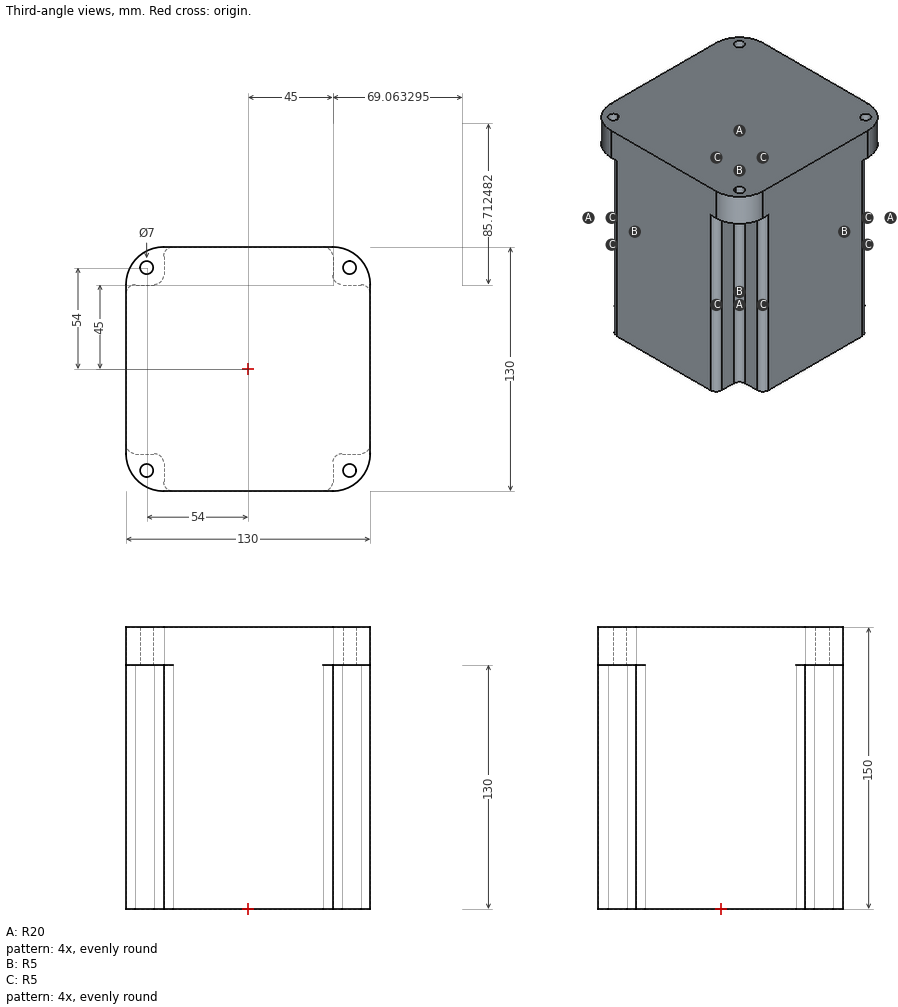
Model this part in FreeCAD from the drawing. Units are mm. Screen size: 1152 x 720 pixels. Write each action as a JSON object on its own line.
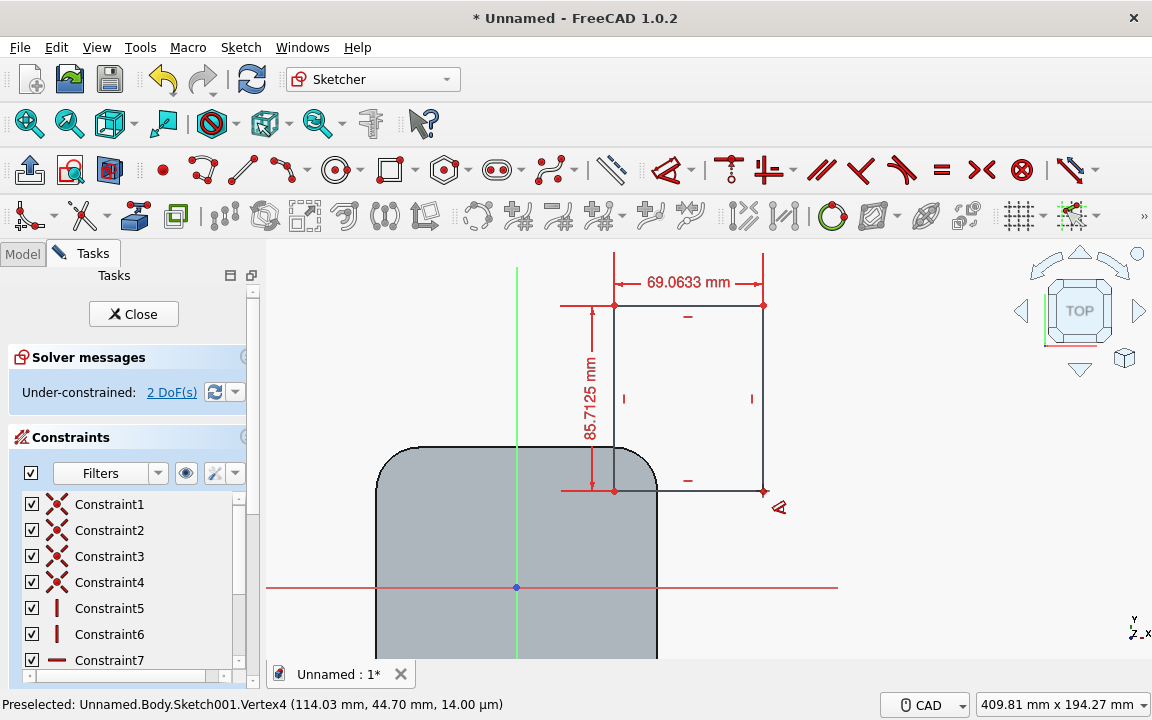
{"action": "left_click", "coordinate": [614, 306]}
{"action": "left_click", "coordinate": [565, 622]}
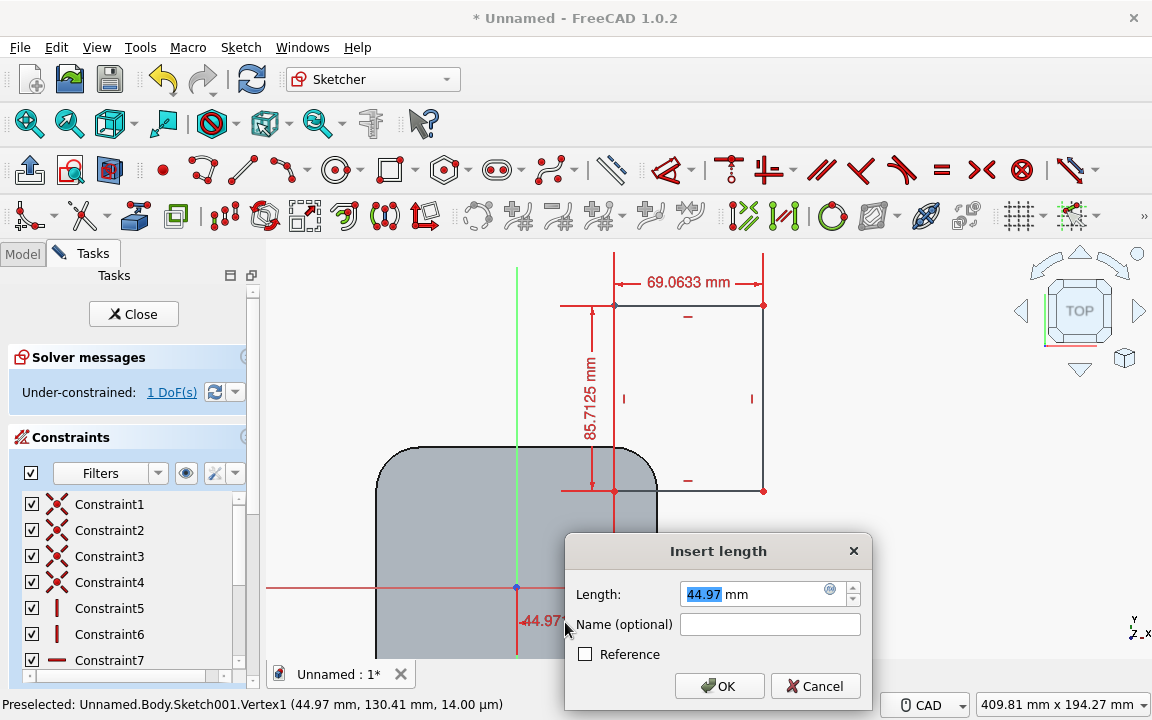
{"action": "type", "text": "45"}
{"action": "key", "text": "Return"}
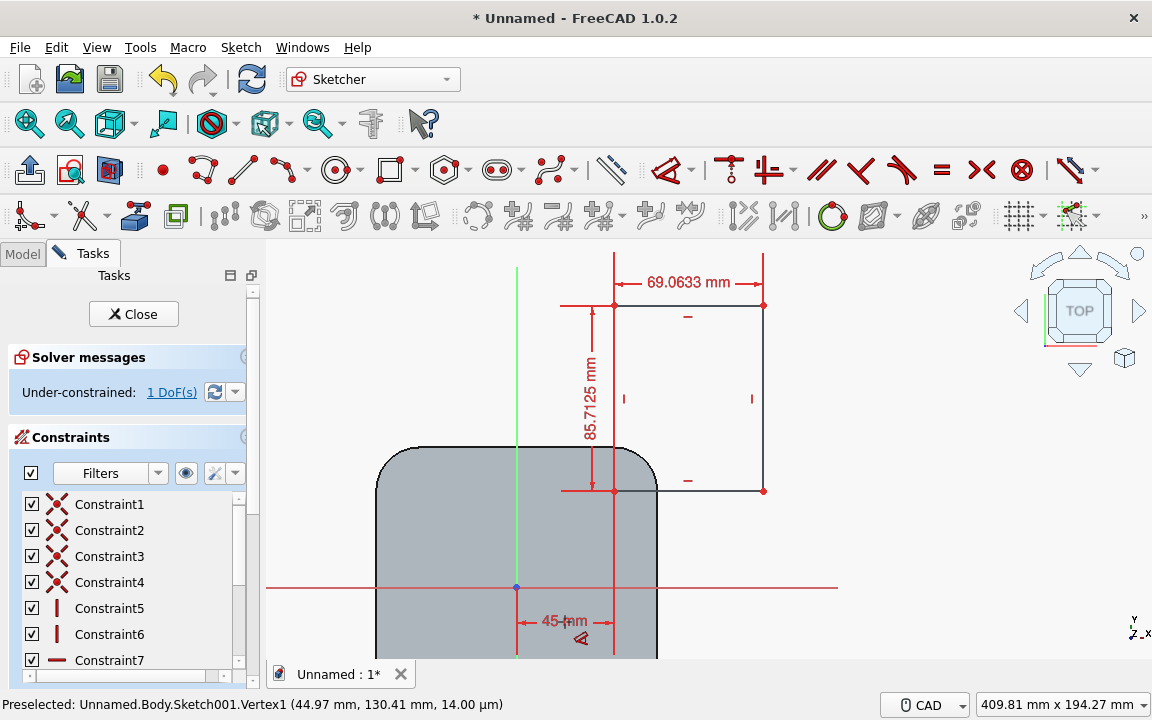
{"action": "left_click", "coordinate": [614, 491]}
{"action": "left_click", "coordinate": [483, 540]}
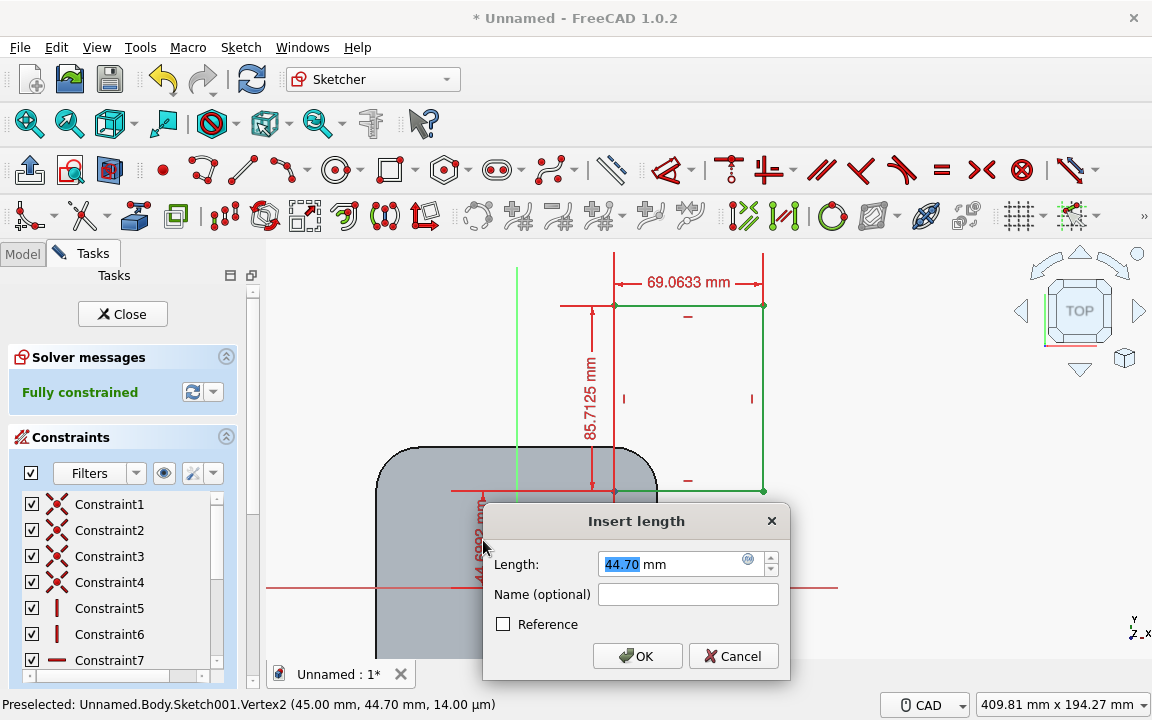
{"action": "type", "text": "45"}
{"action": "key", "text": "Return"}
{"action": "key", "text": "Escape"}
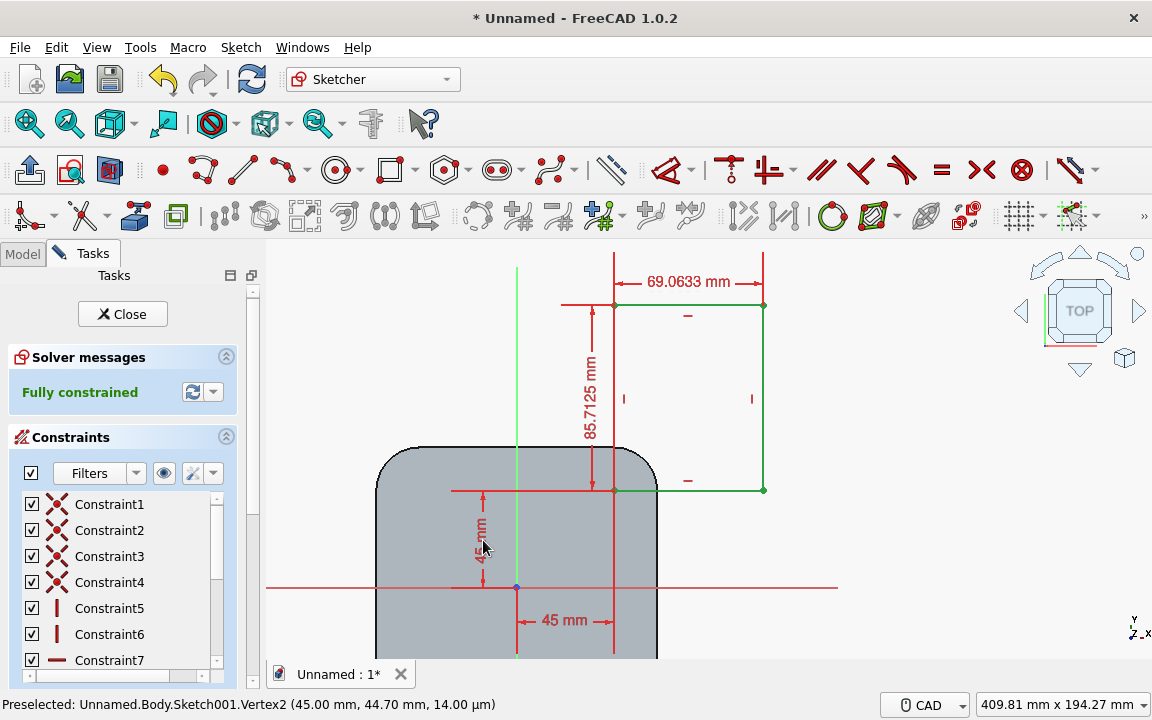
{"action": "left_click", "coordinate": [123, 314]}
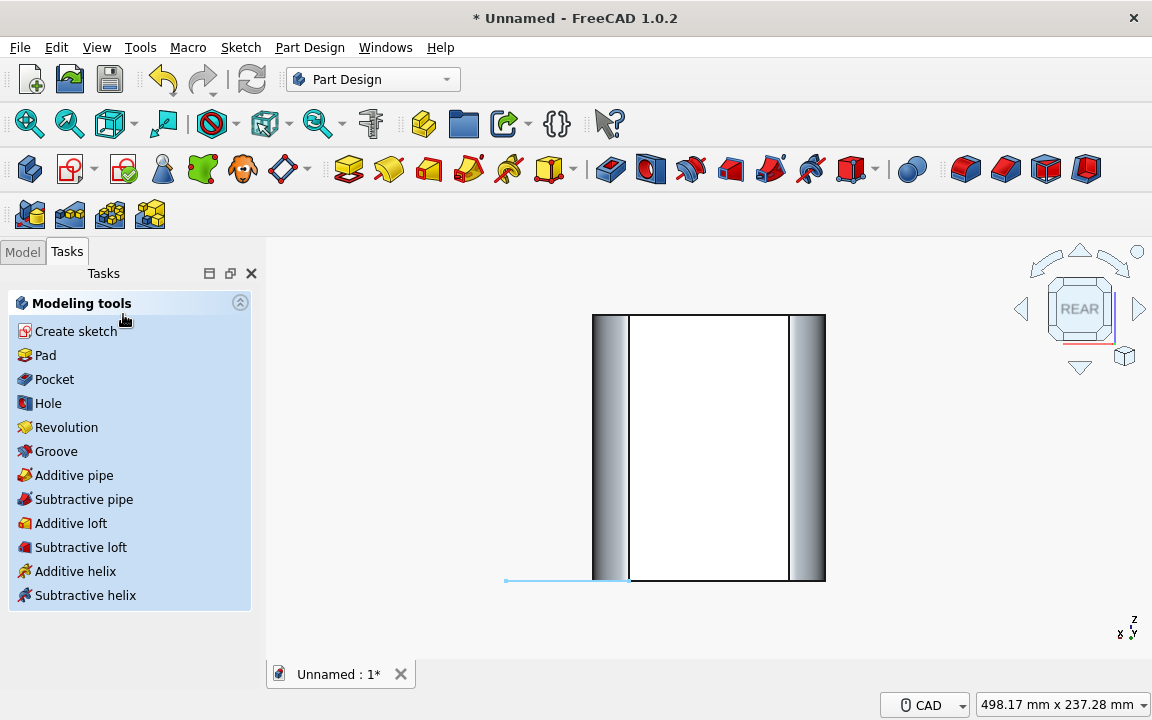
{"action": "left_click", "coordinate": [612, 170]}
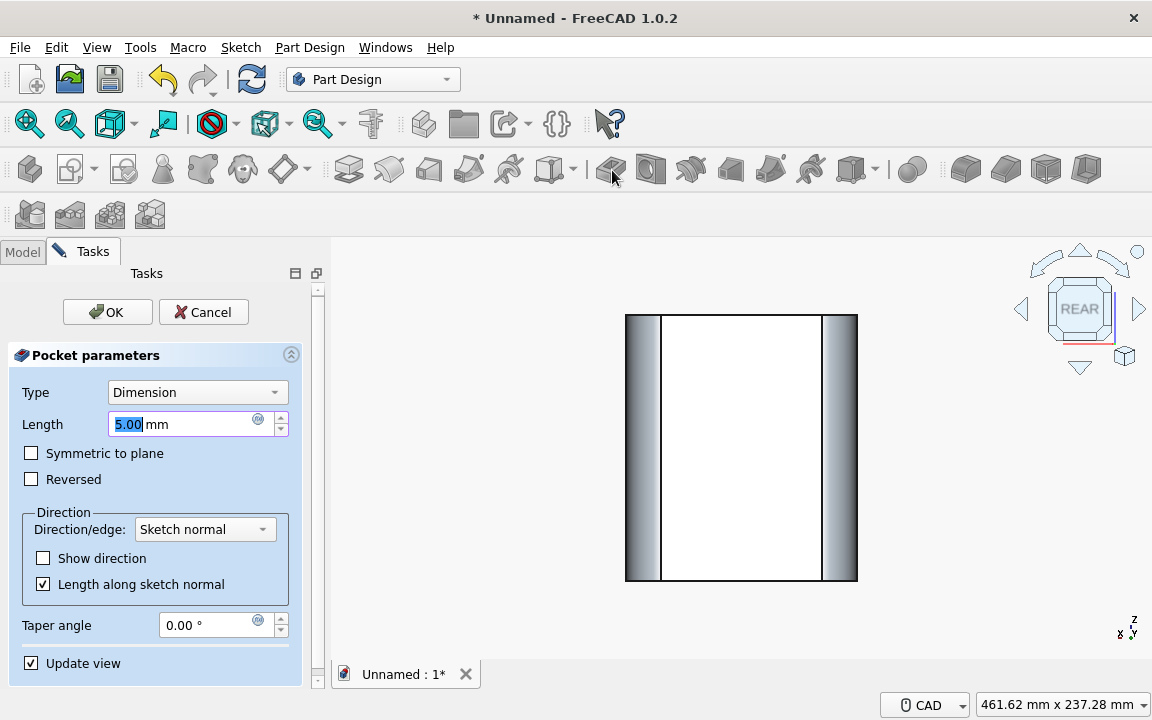
{"action": "type", "text": "130"}
{"action": "key", "text": "Tab"}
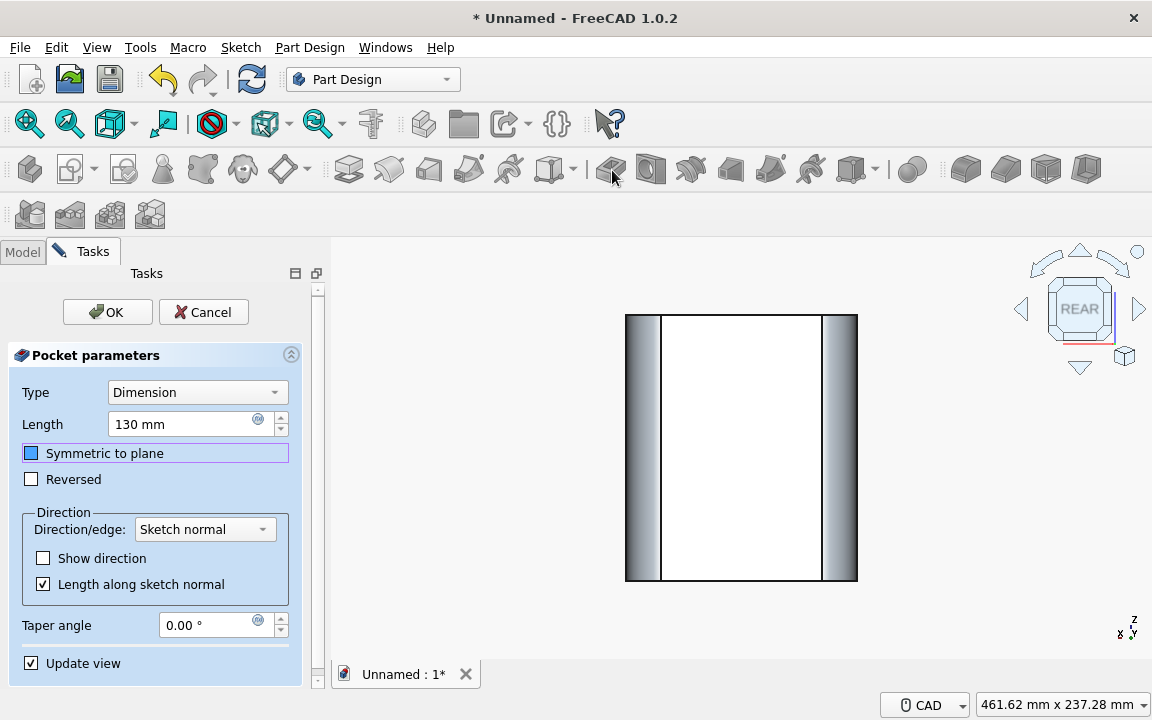
{"action": "left_click", "coordinate": [30, 479]}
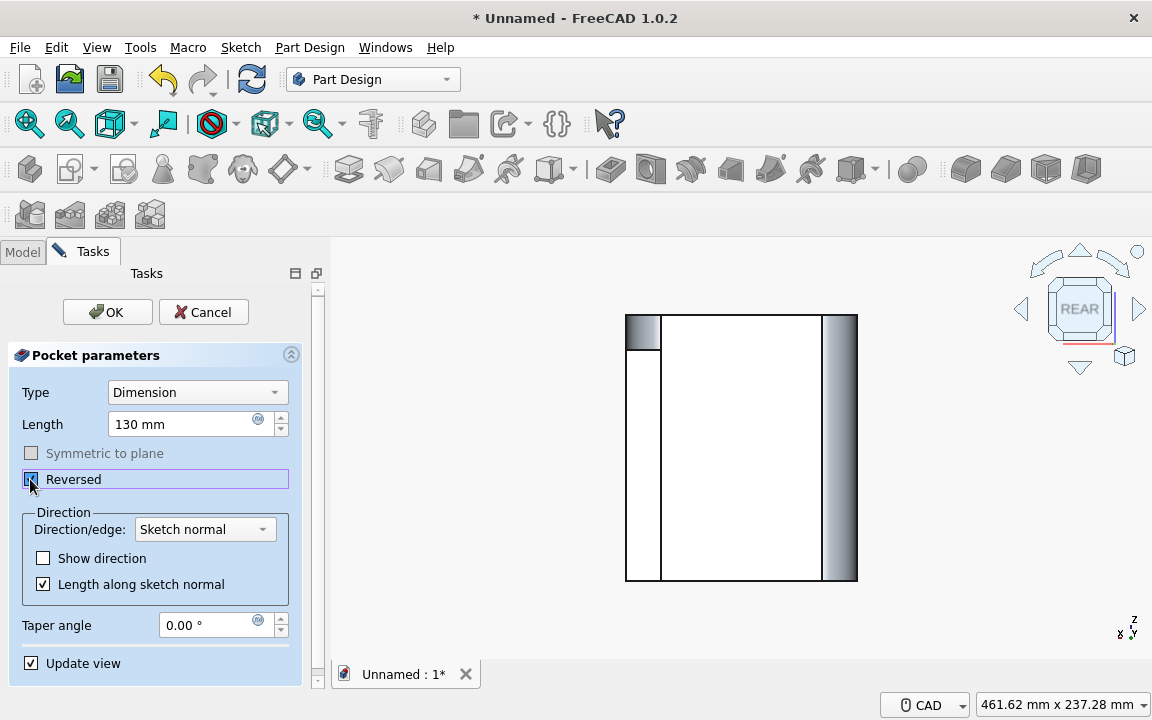
{"action": "left_click", "coordinate": [108, 312]}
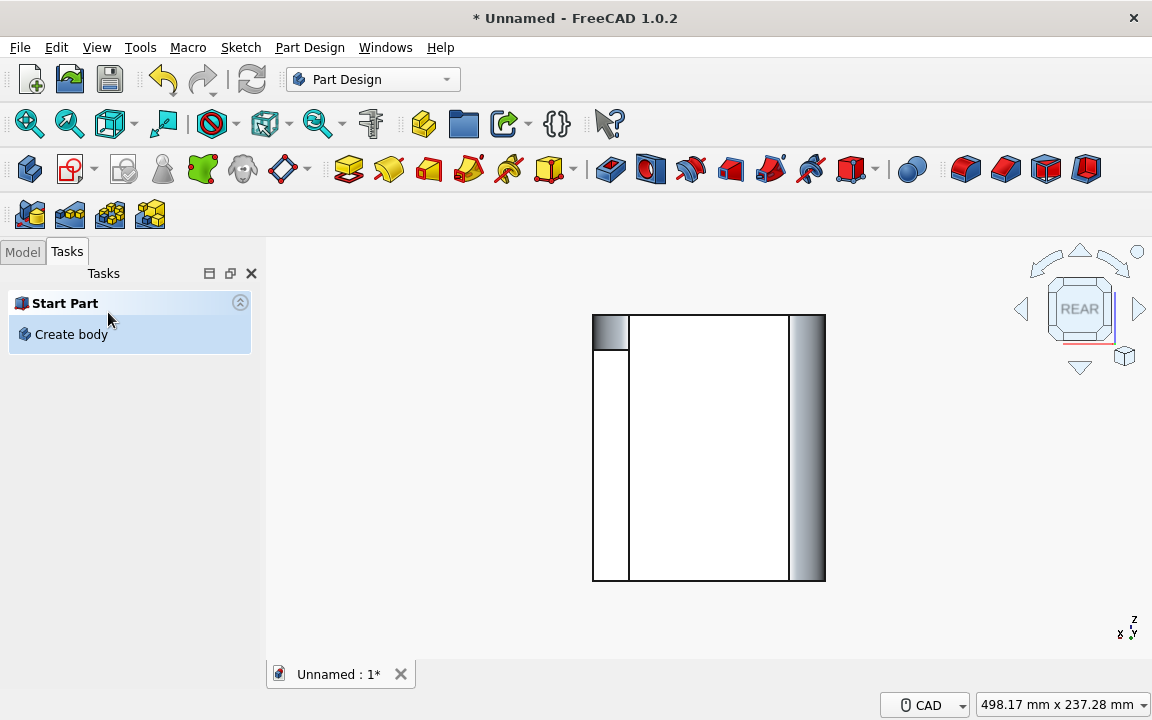
{"action": "left_click", "coordinate": [23, 251]}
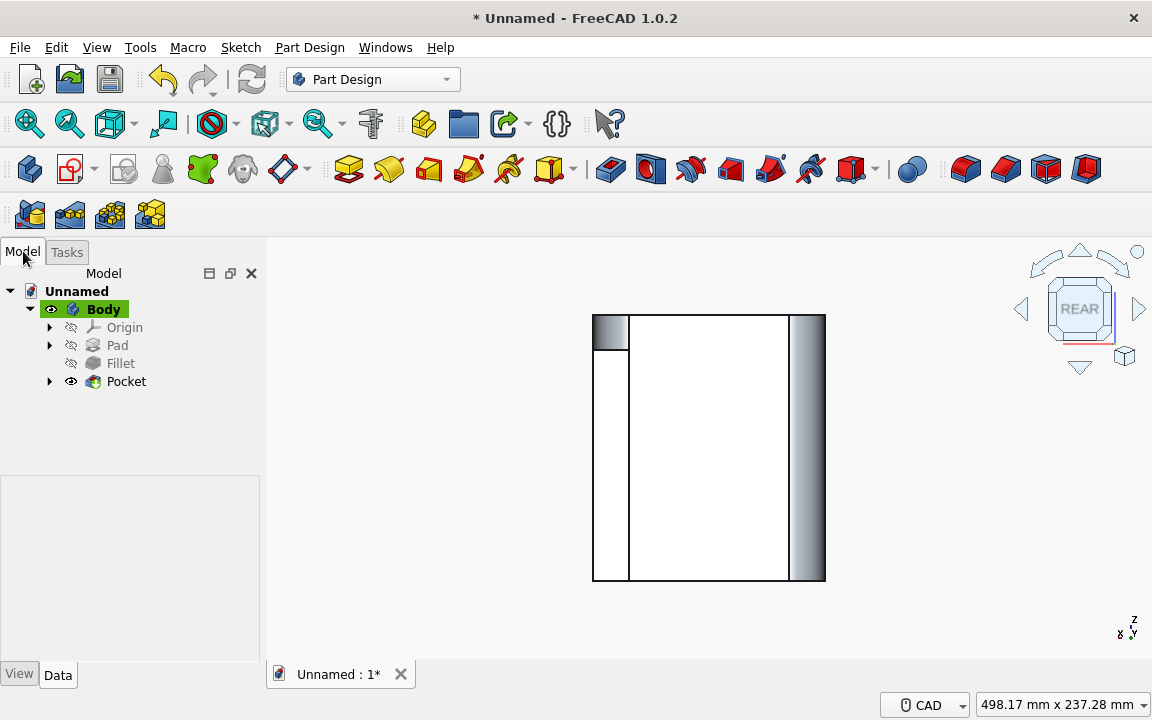
{"action": "left_click", "coordinate": [116, 381]}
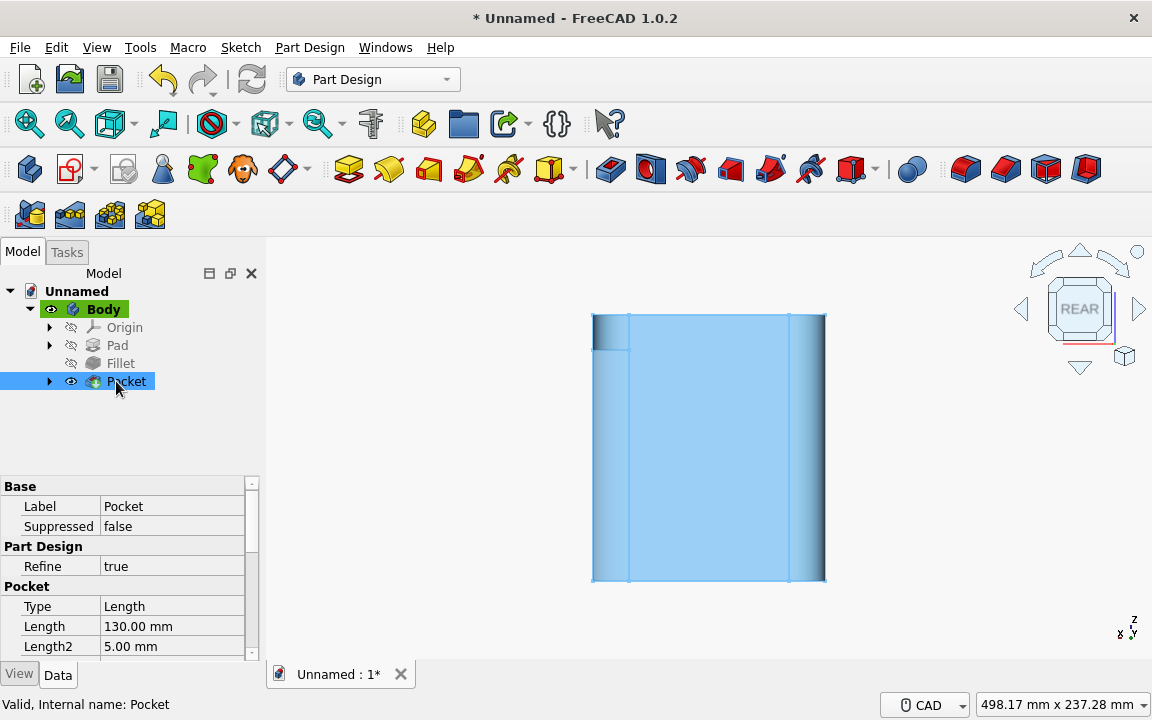
{"action": "left_click", "coordinate": [110, 214]}